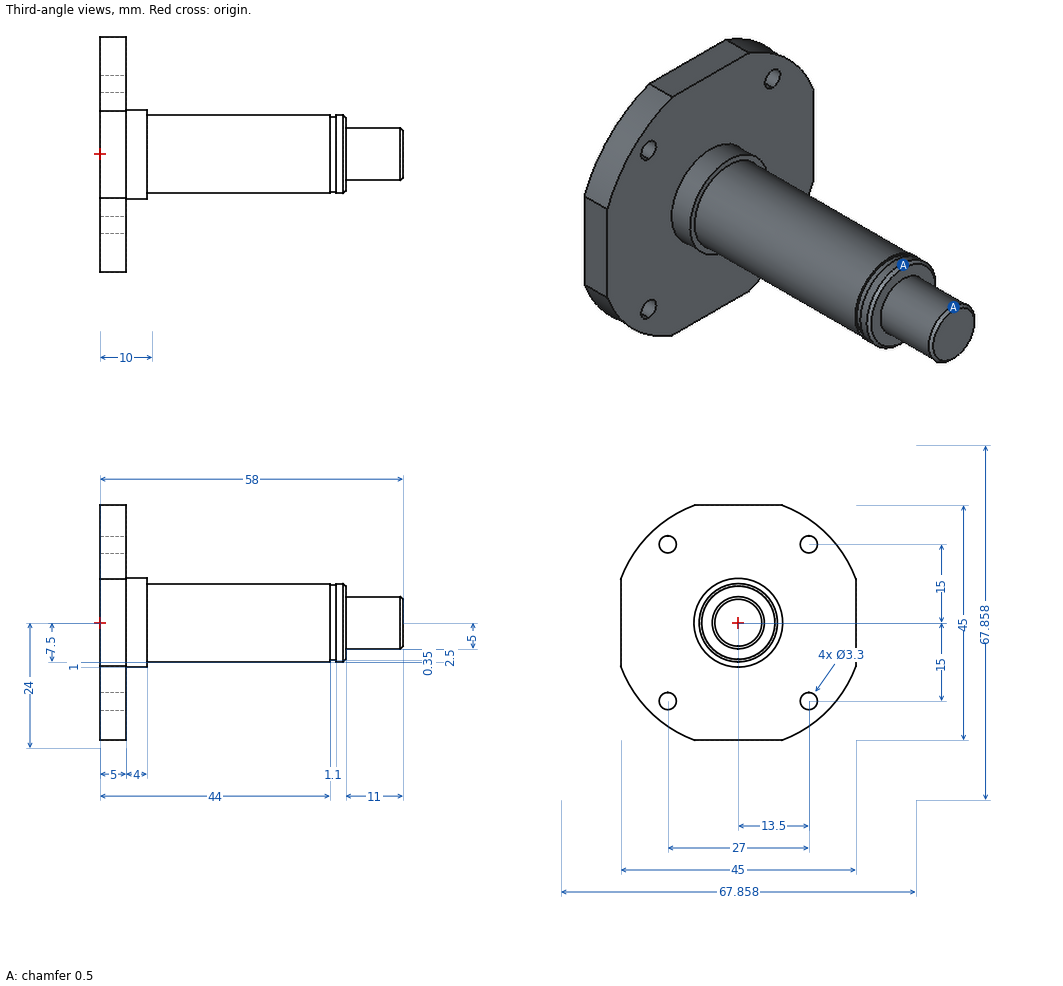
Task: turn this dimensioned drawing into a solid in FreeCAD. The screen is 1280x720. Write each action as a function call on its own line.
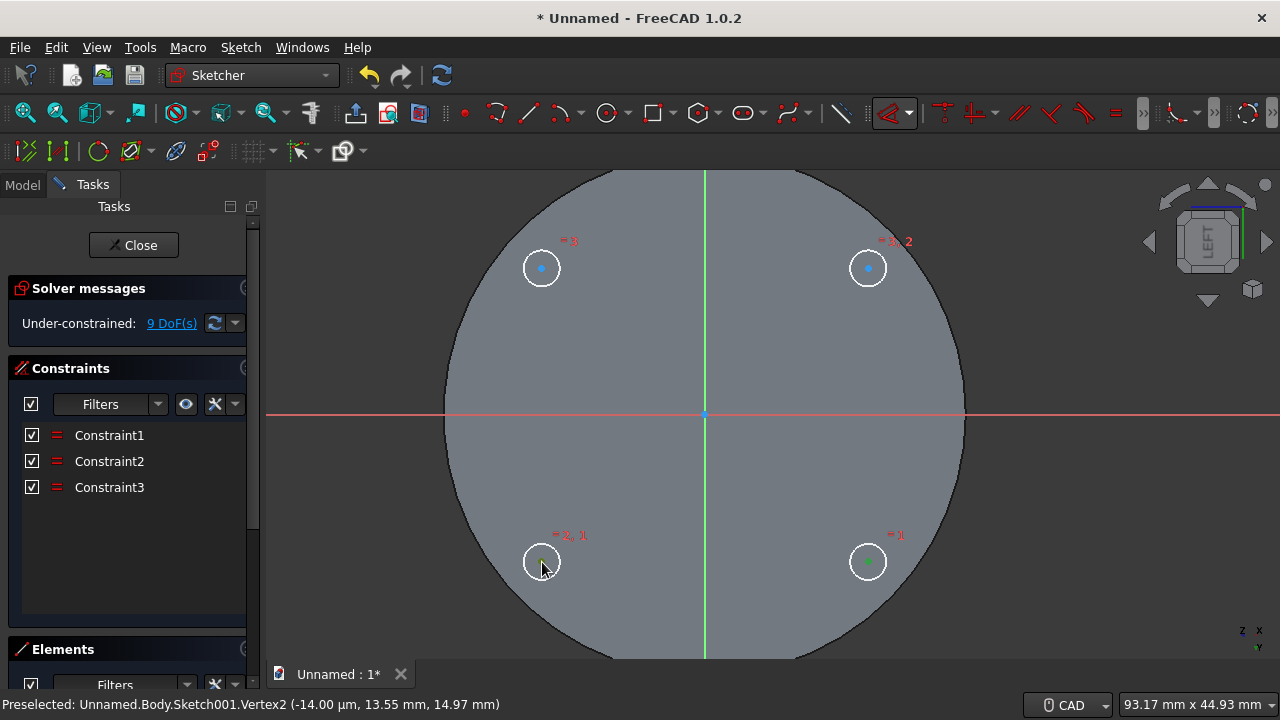
click(998, 114)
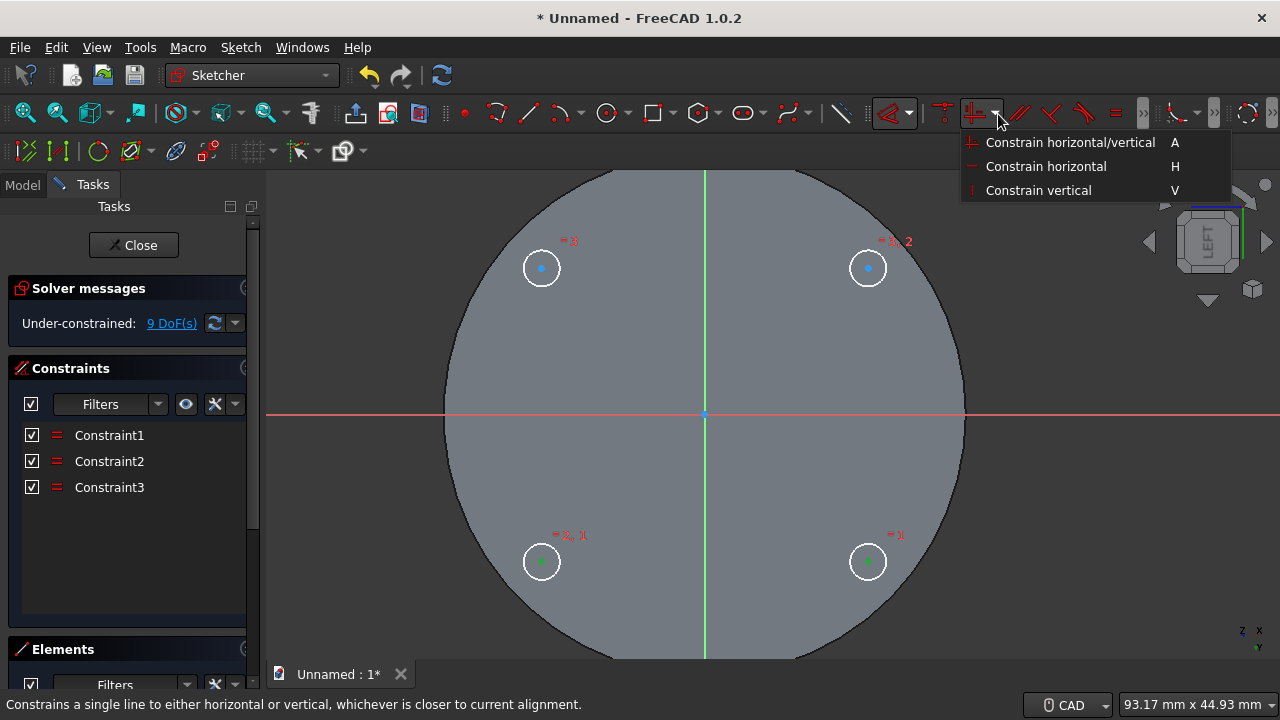
click(1096, 166)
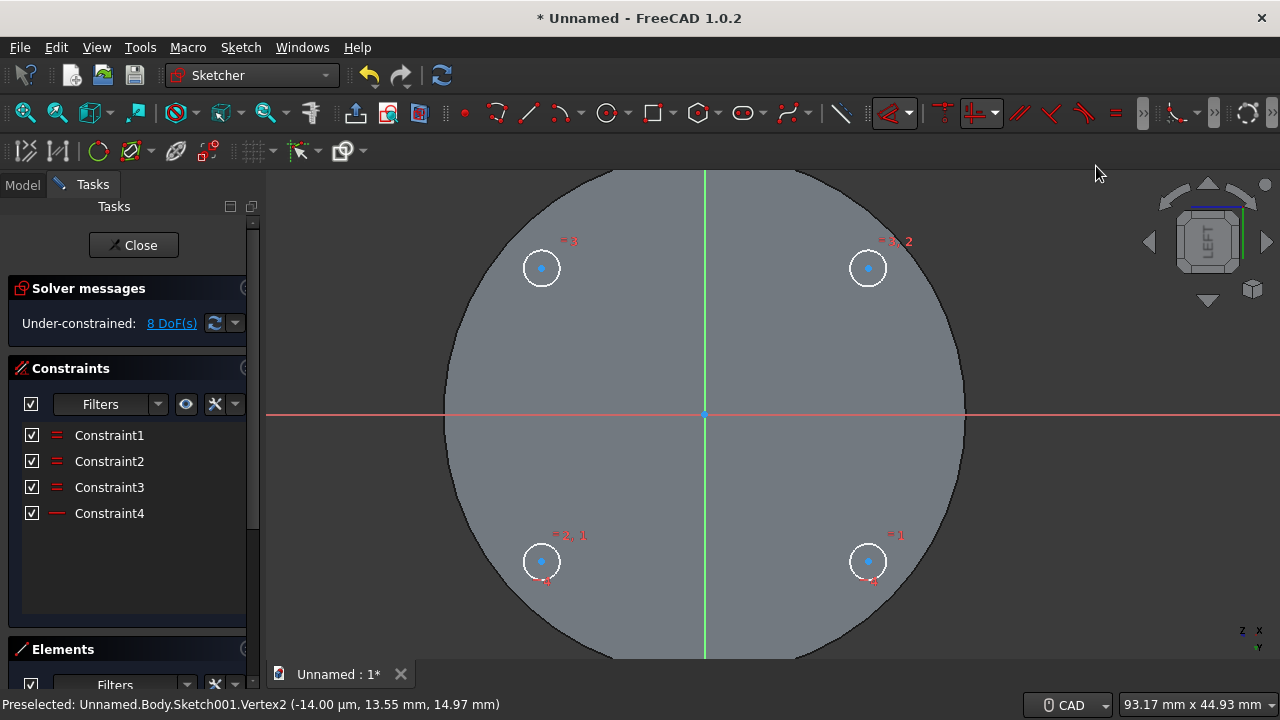
click(868, 562)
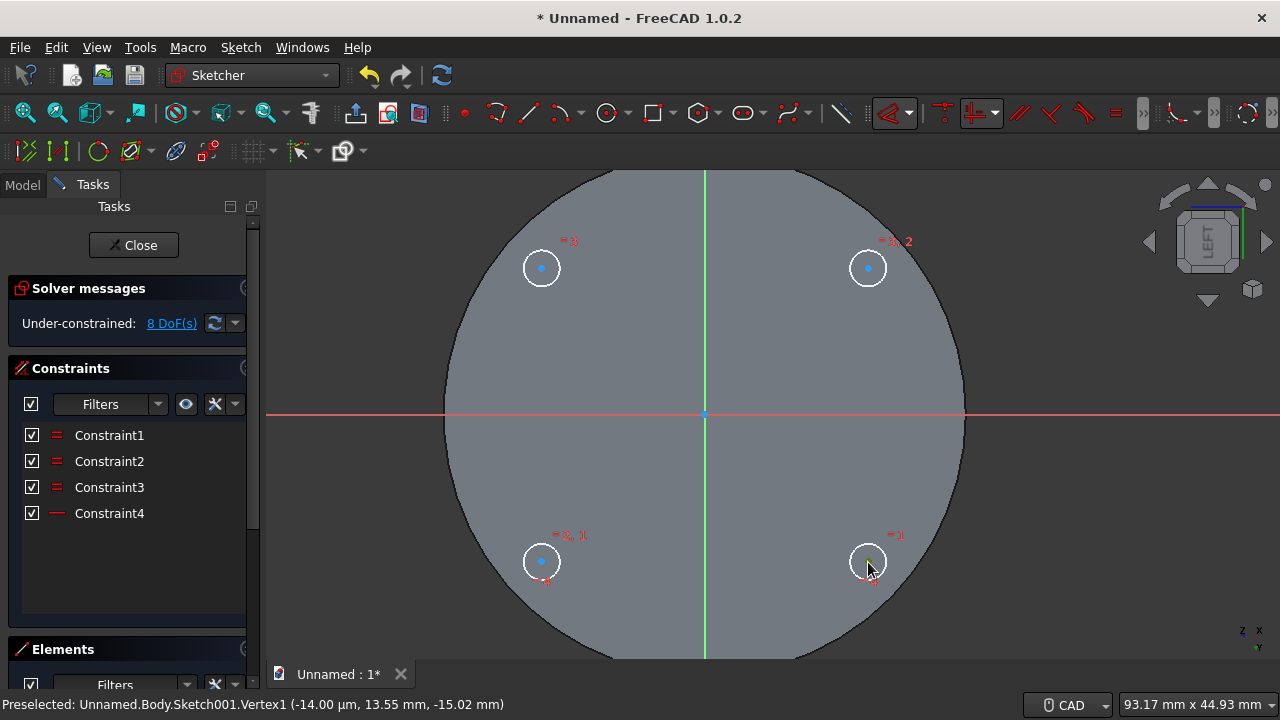
click(868, 268)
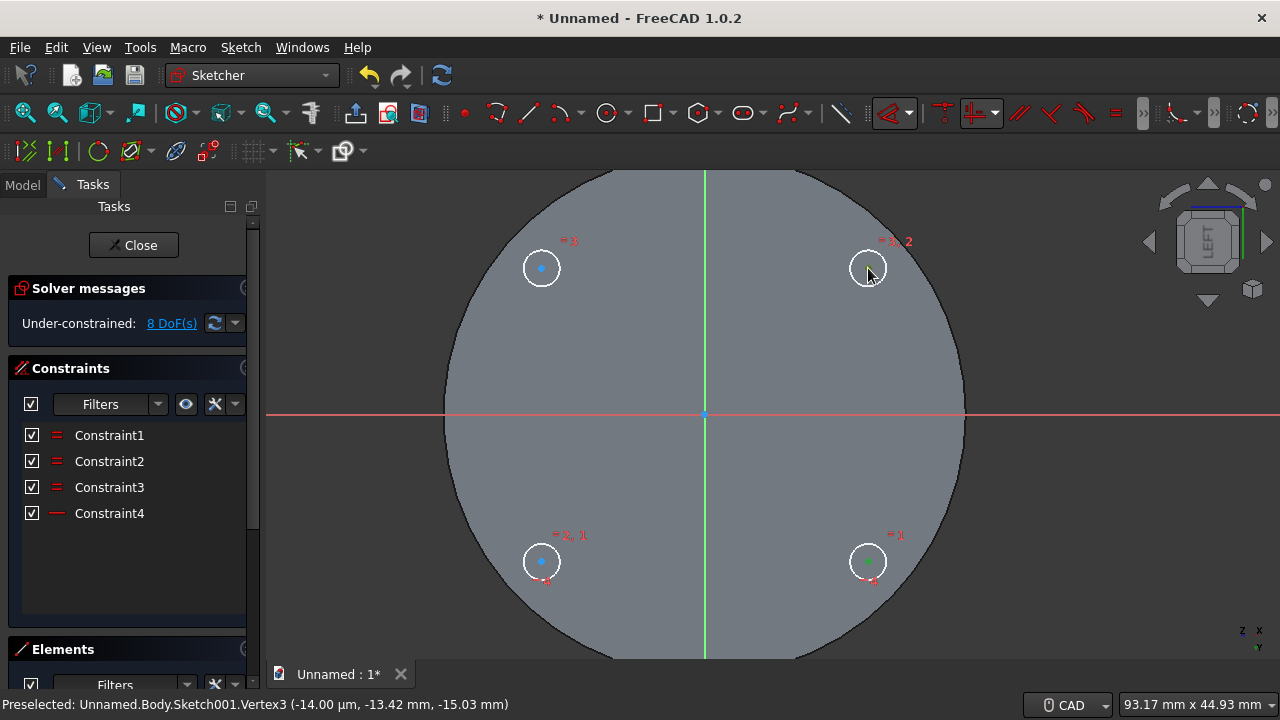
click(998, 114)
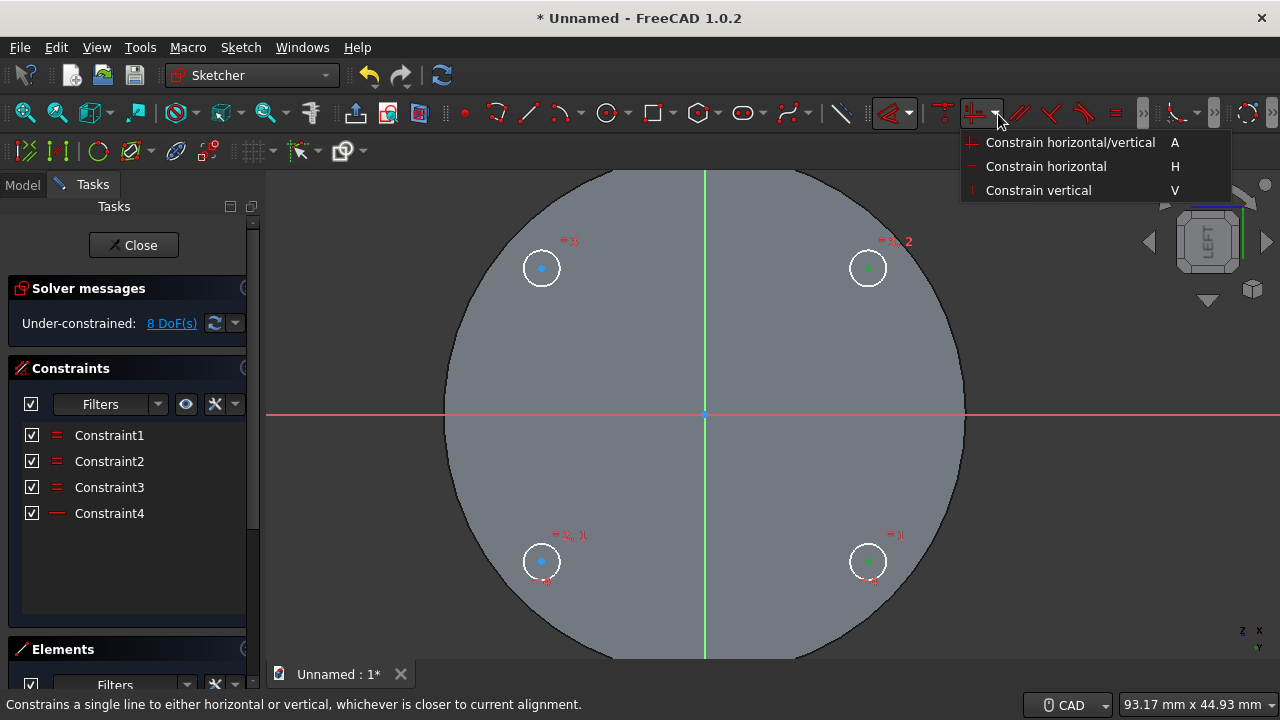
click(1096, 190)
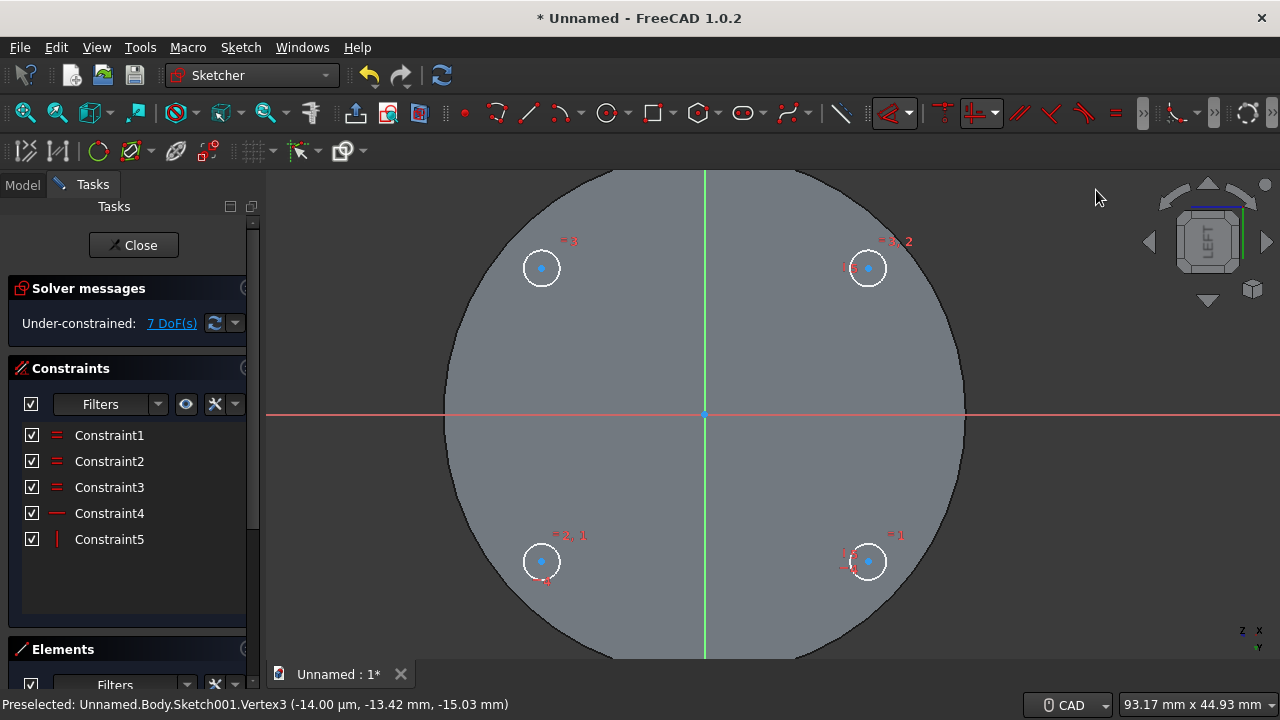
click(542, 562)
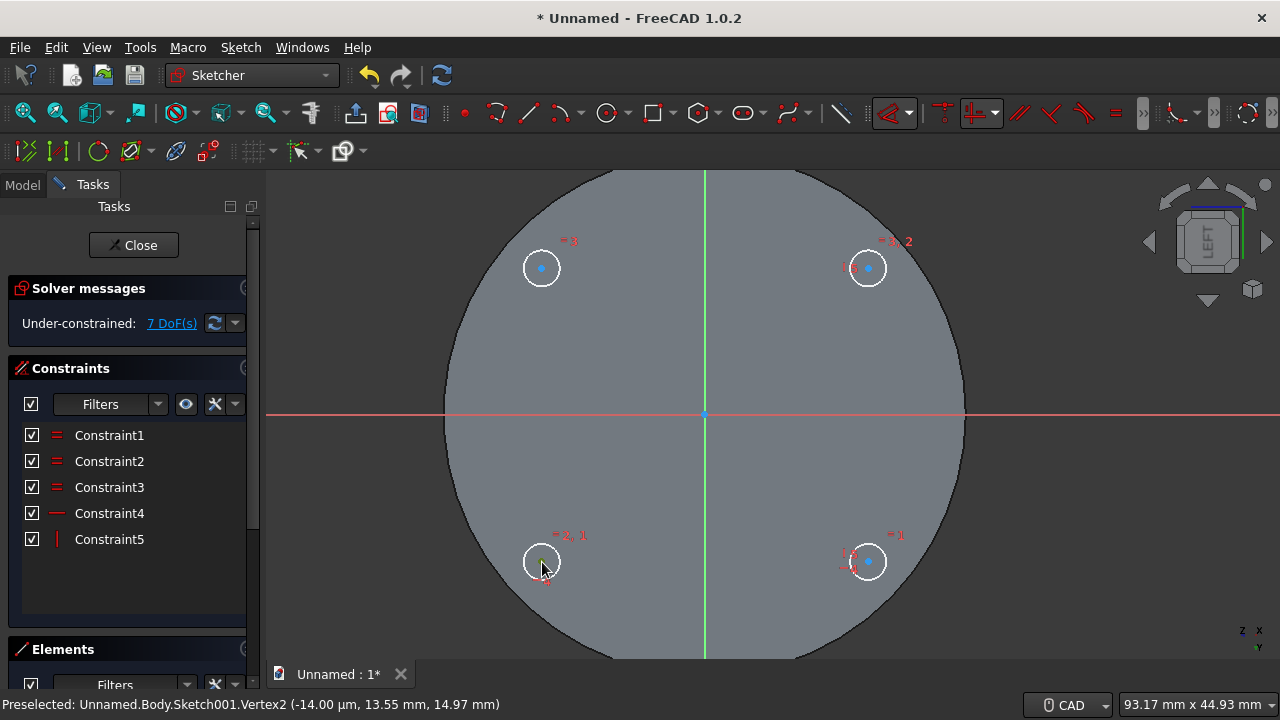
click(542, 268)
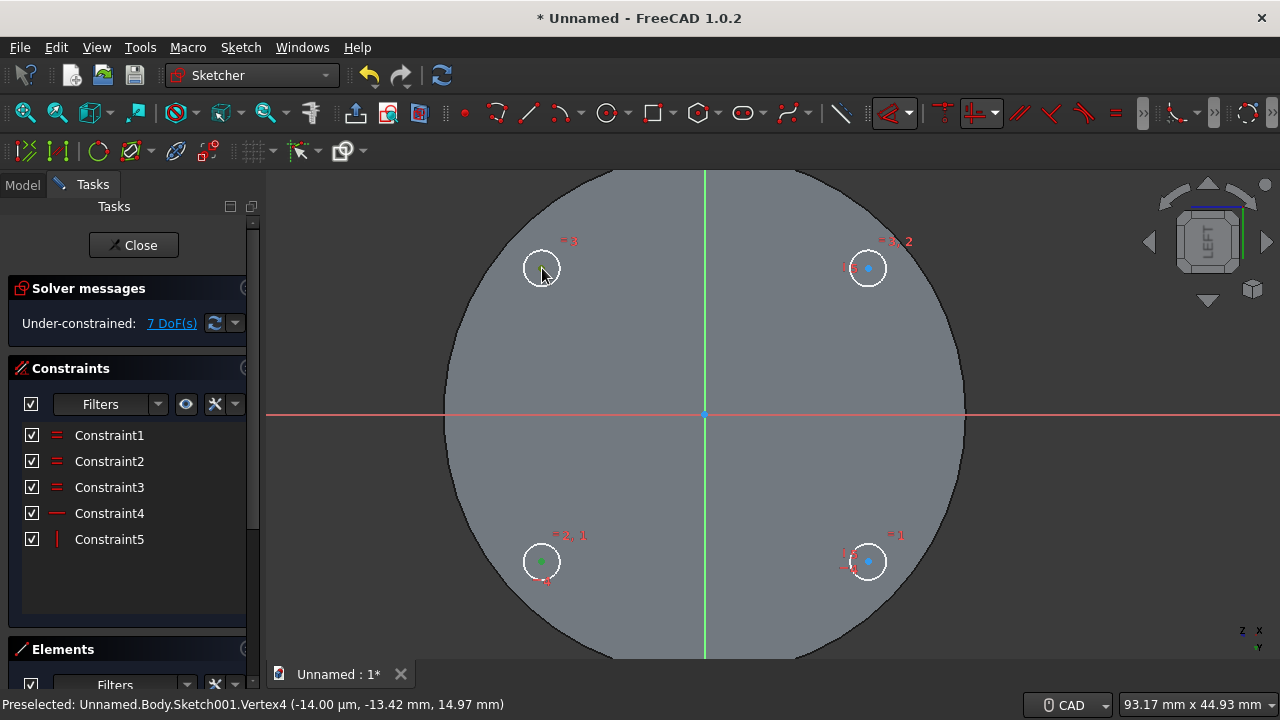
key(v)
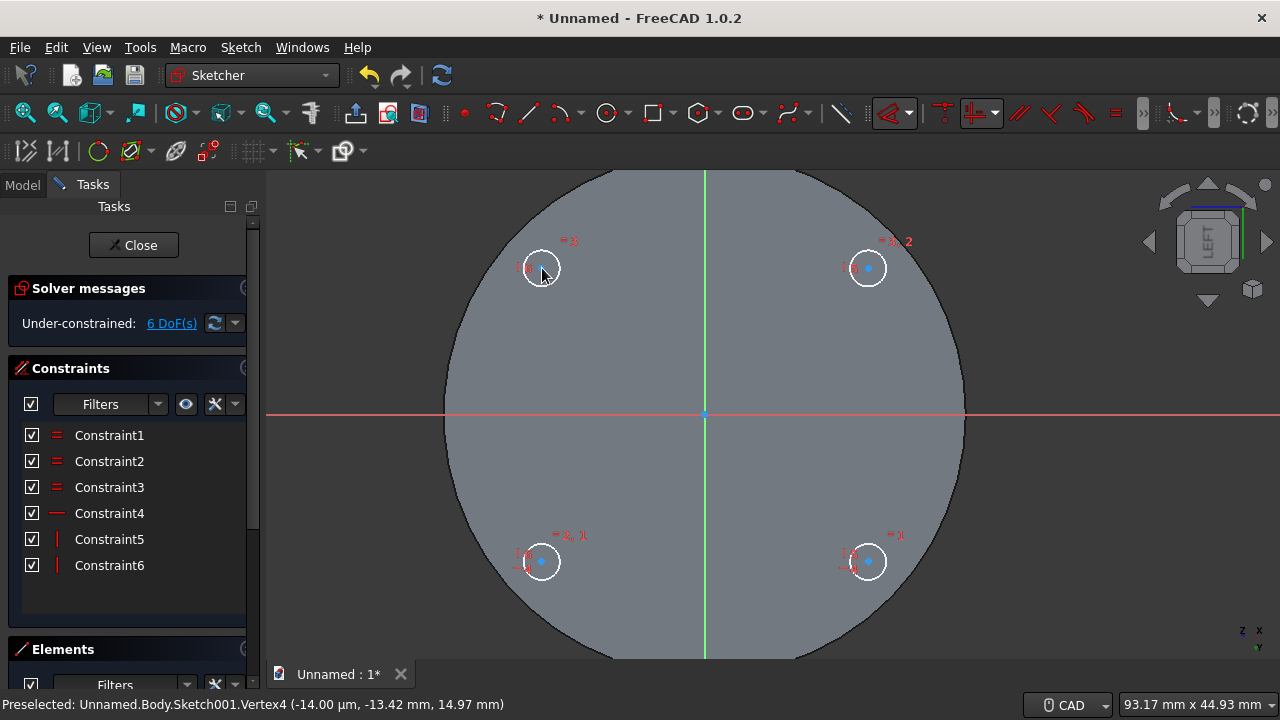
click(868, 268)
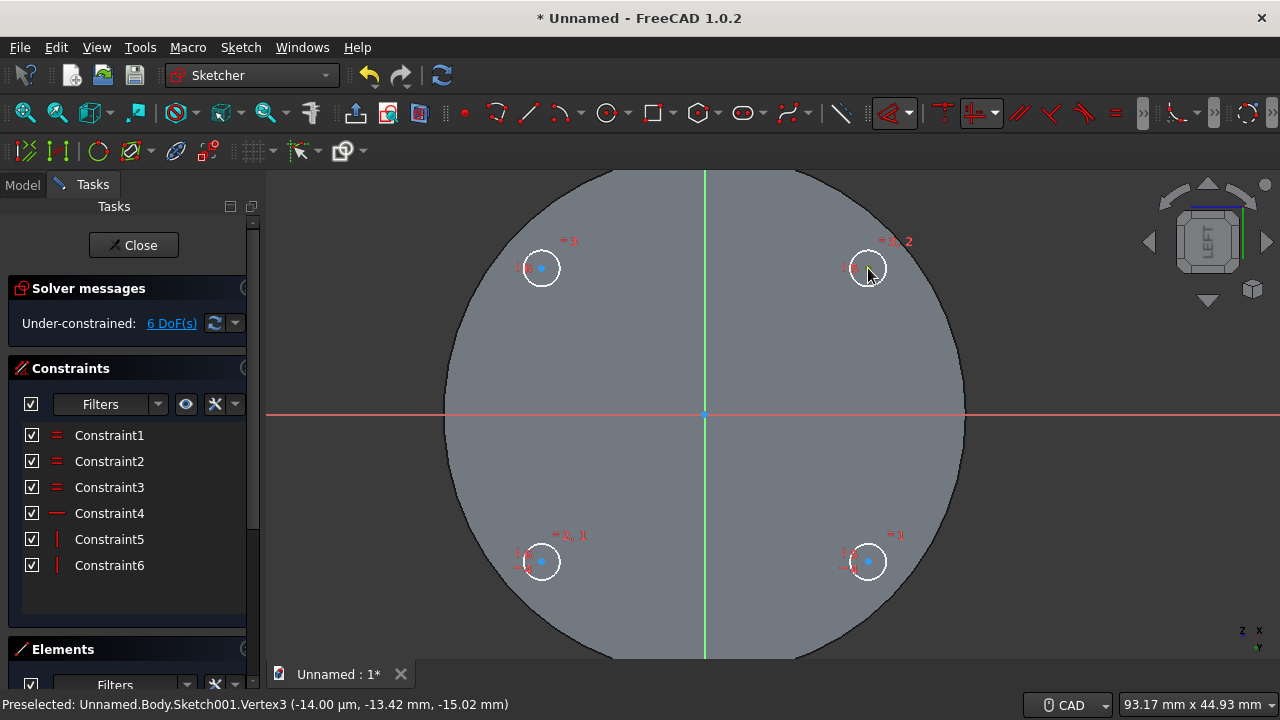
click(542, 268)